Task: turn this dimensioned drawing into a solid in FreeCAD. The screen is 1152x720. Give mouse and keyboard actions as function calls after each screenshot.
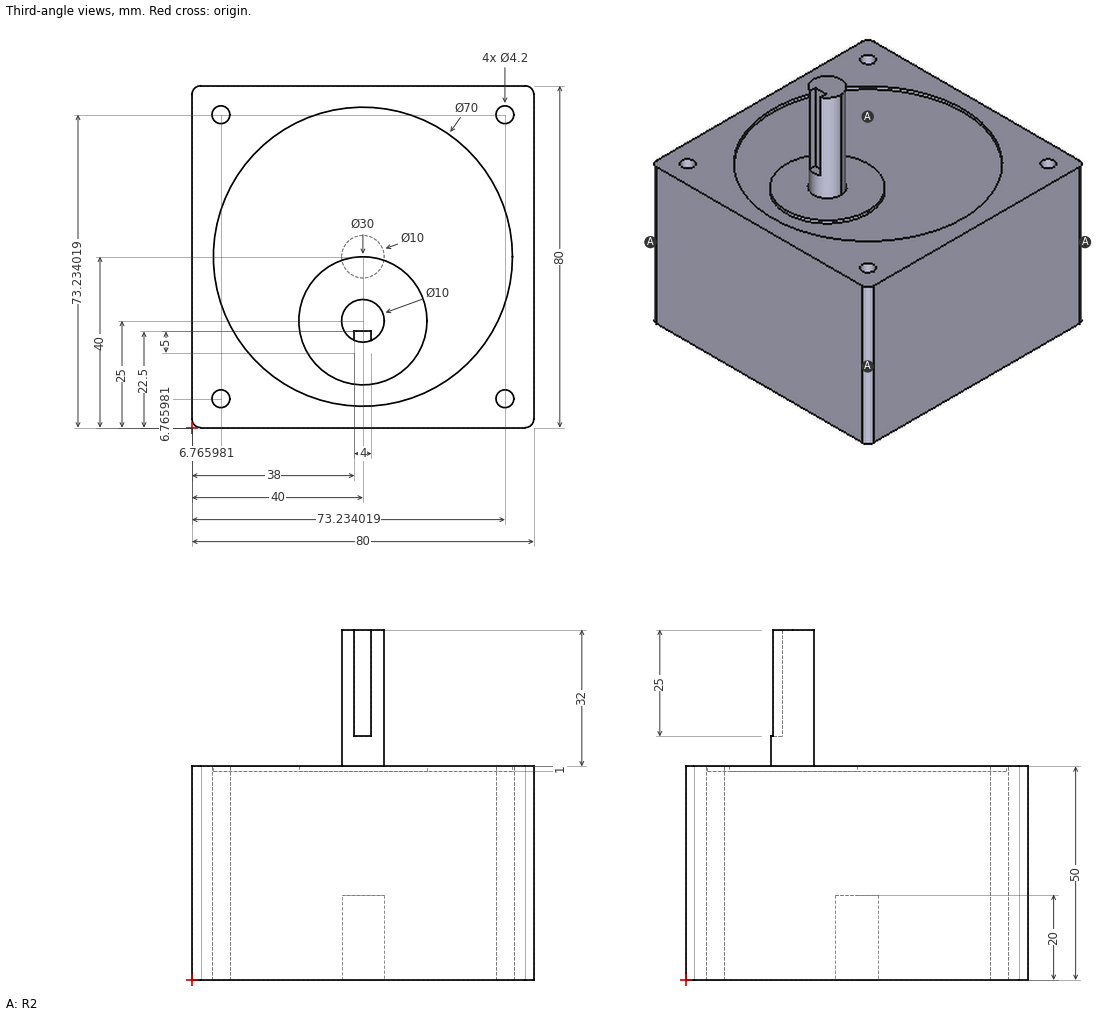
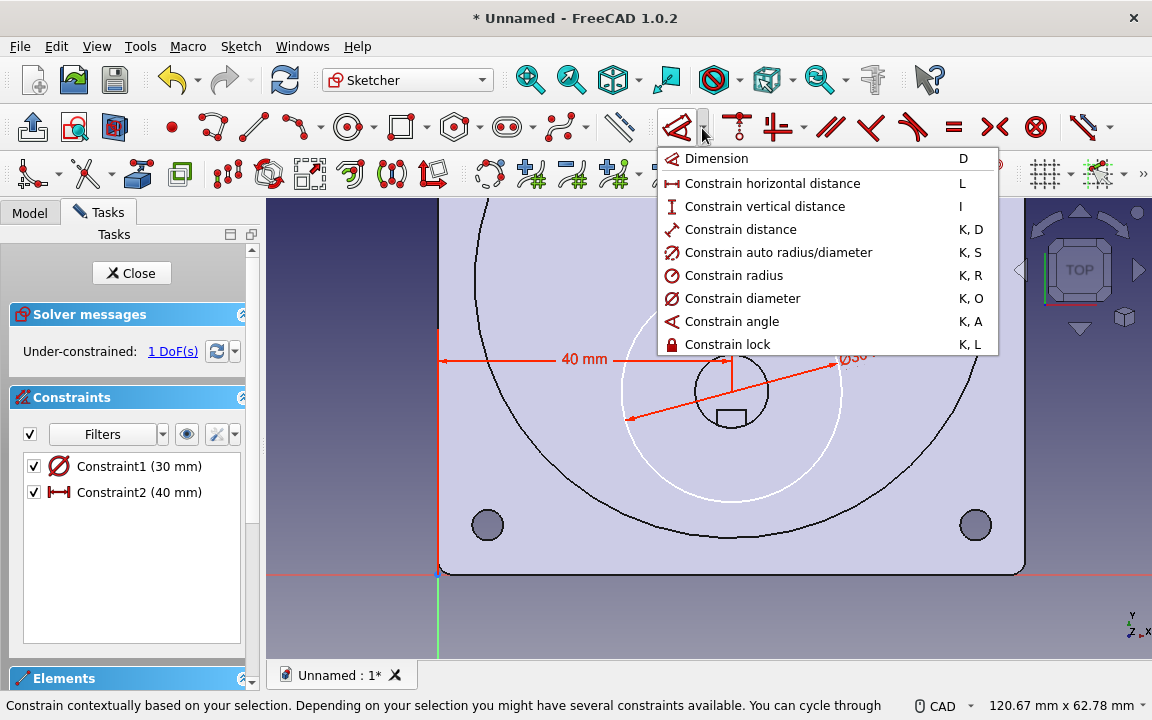
click(828, 206)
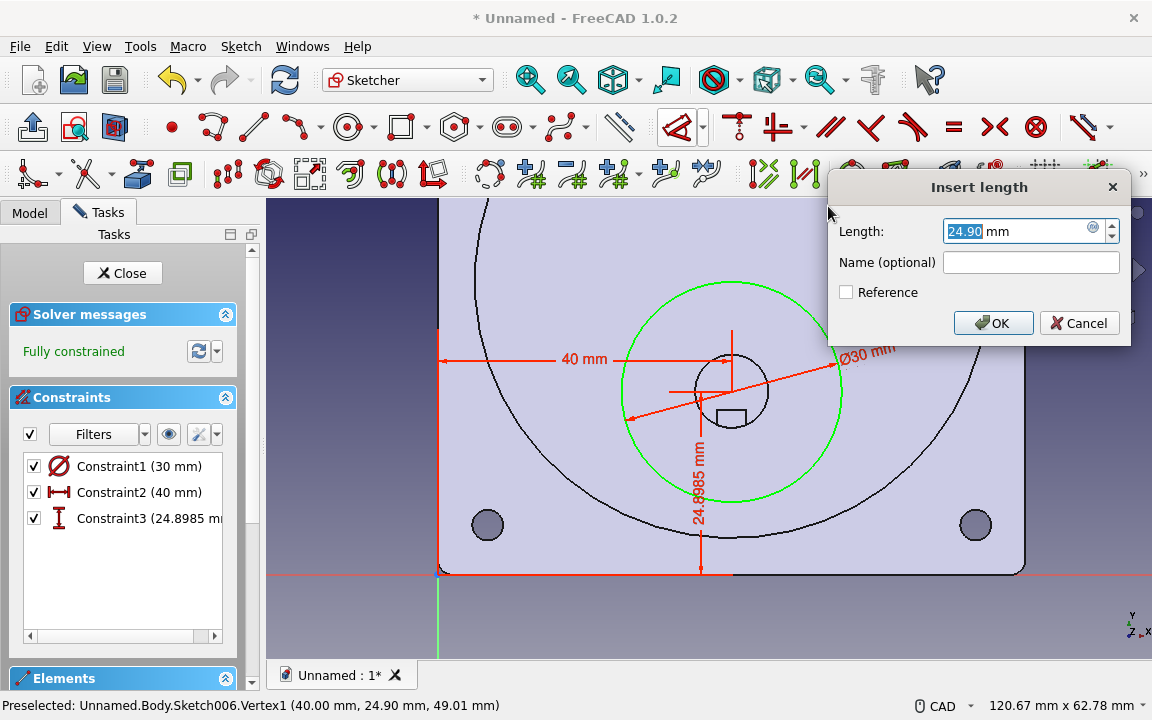
text(25)
key(Return)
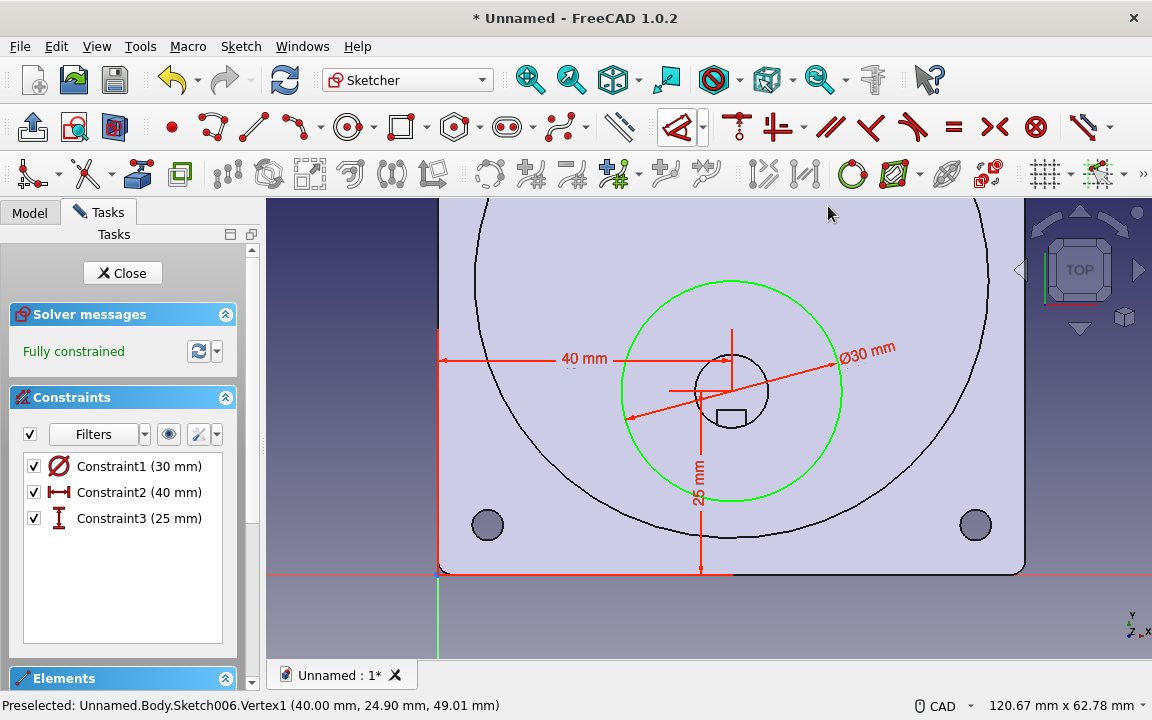
click(123, 273)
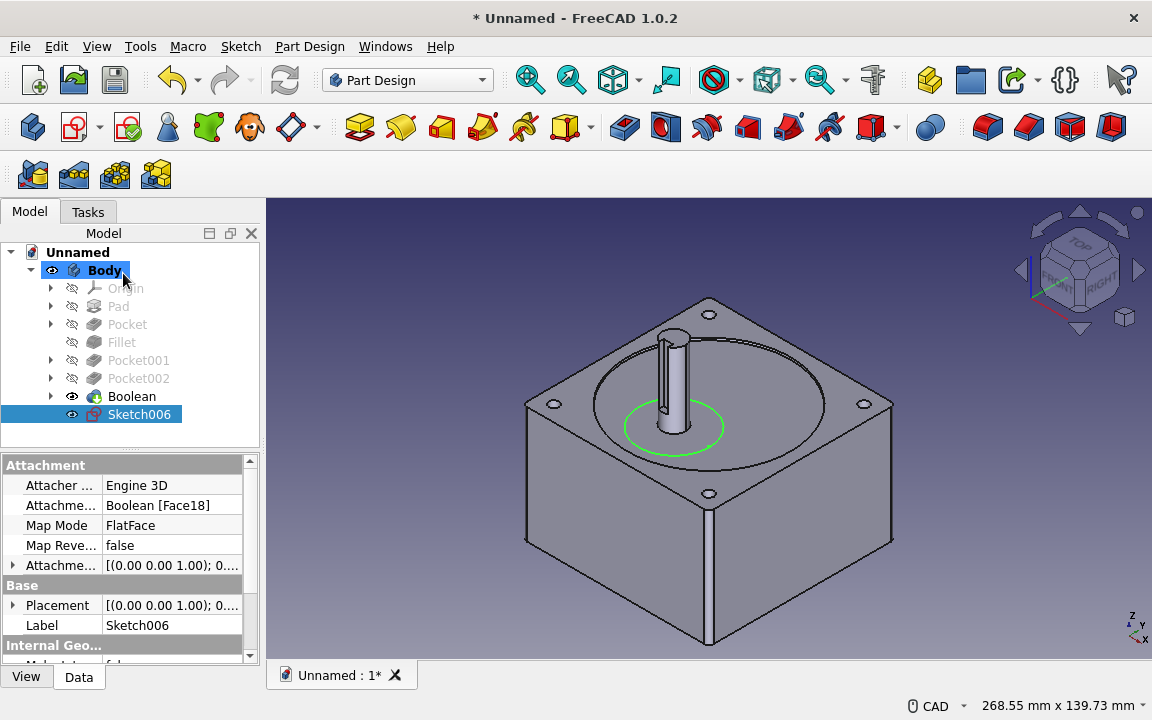
click(360, 128)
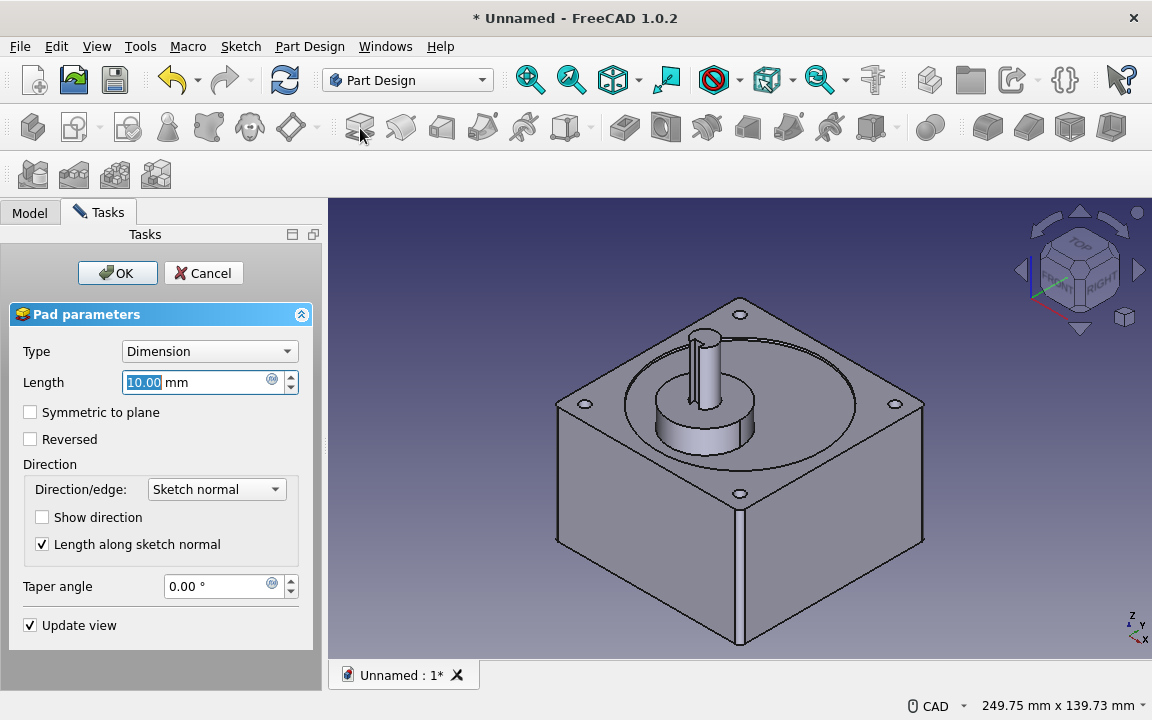
text(1)
key(Tab)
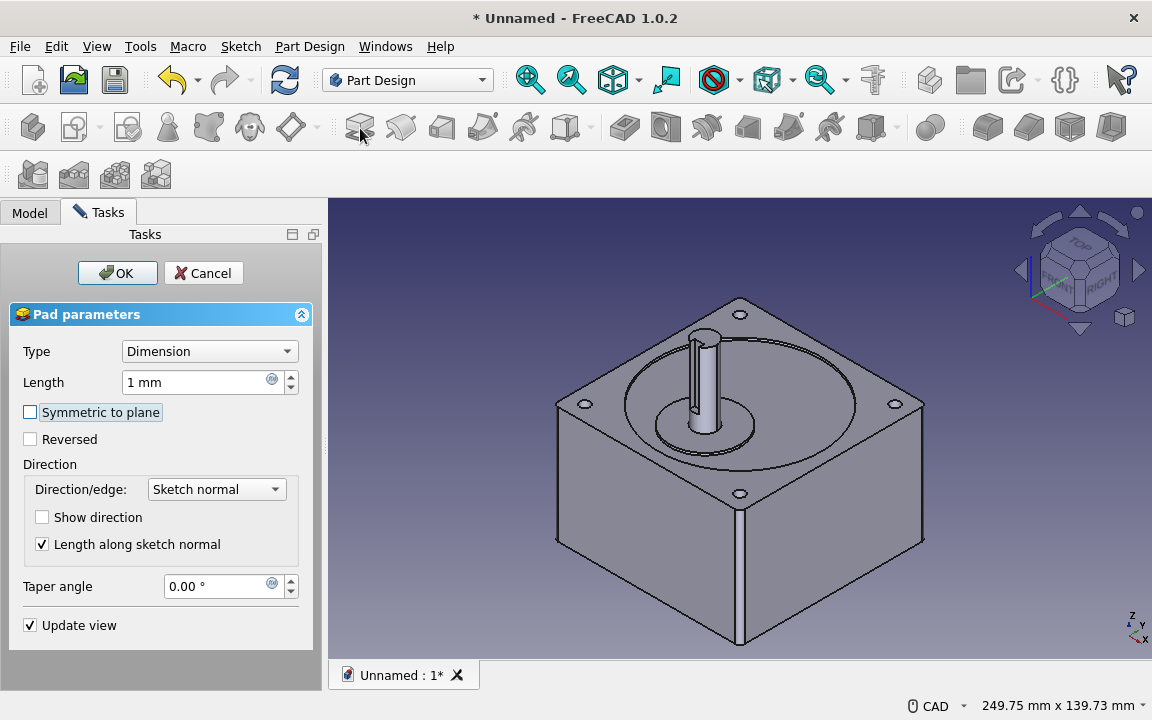
click(118, 273)